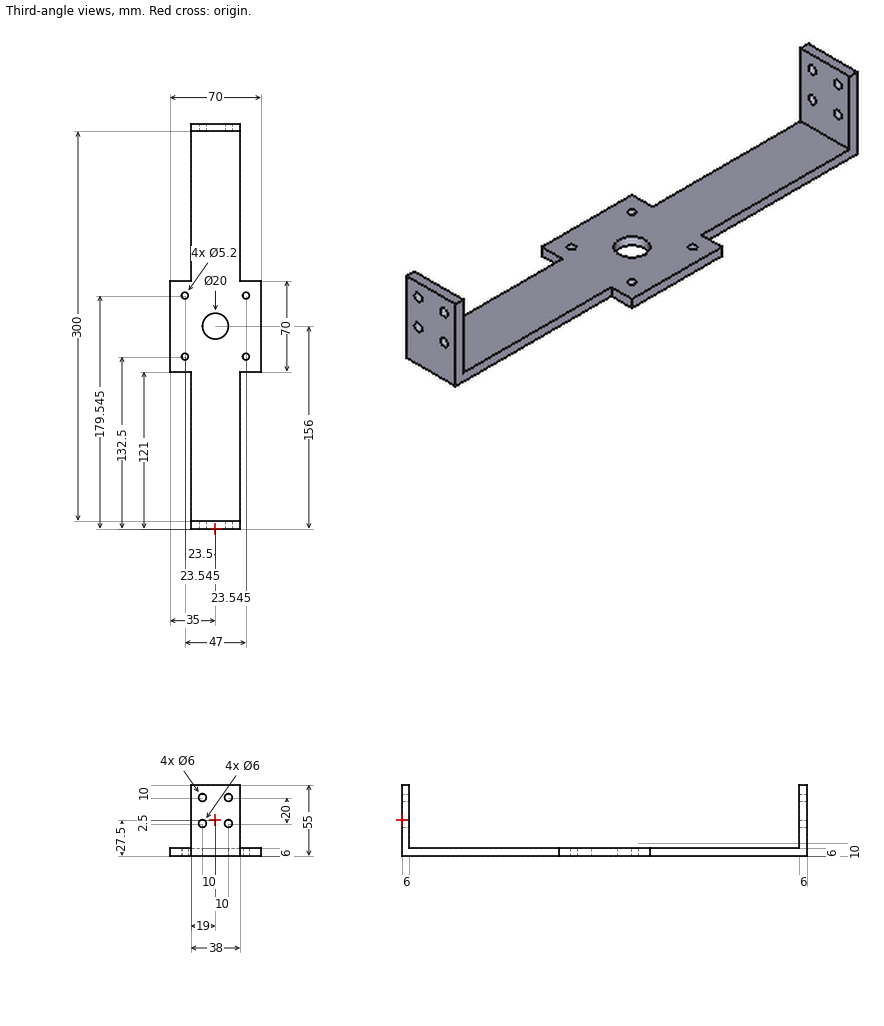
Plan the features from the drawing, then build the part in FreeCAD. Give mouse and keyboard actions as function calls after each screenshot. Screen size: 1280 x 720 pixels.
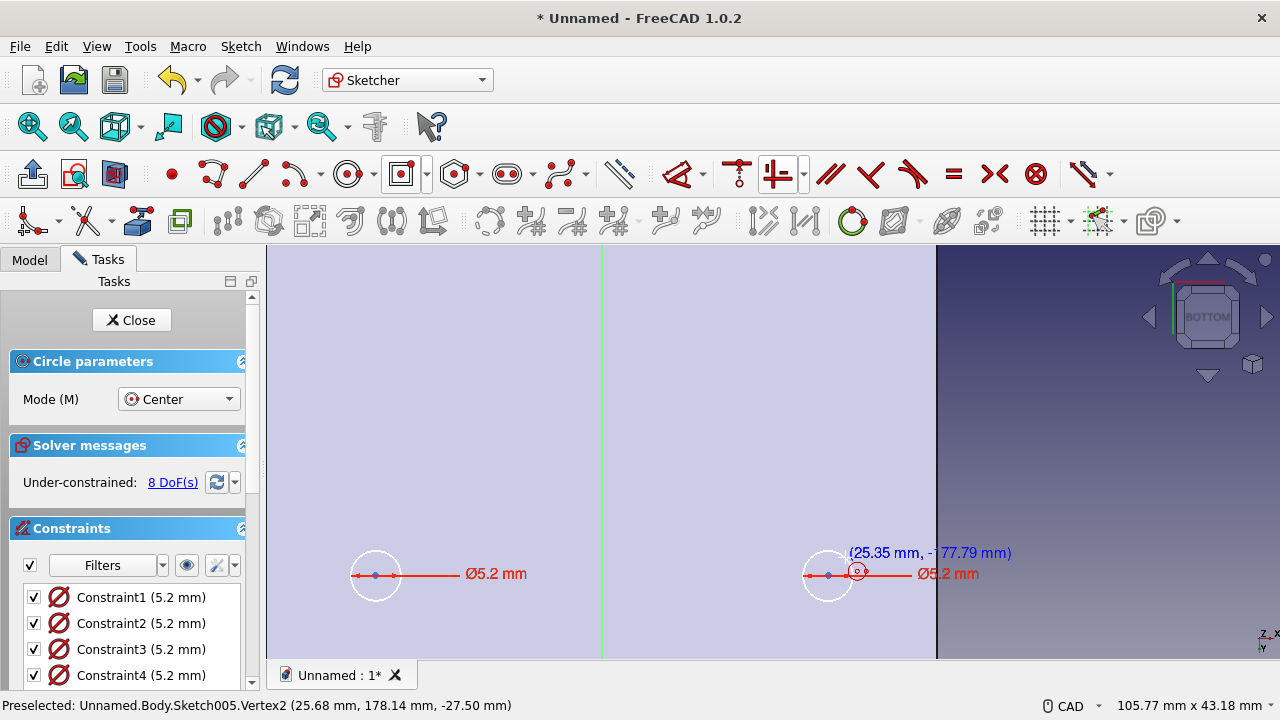
click(602, 349)
move(670, 281)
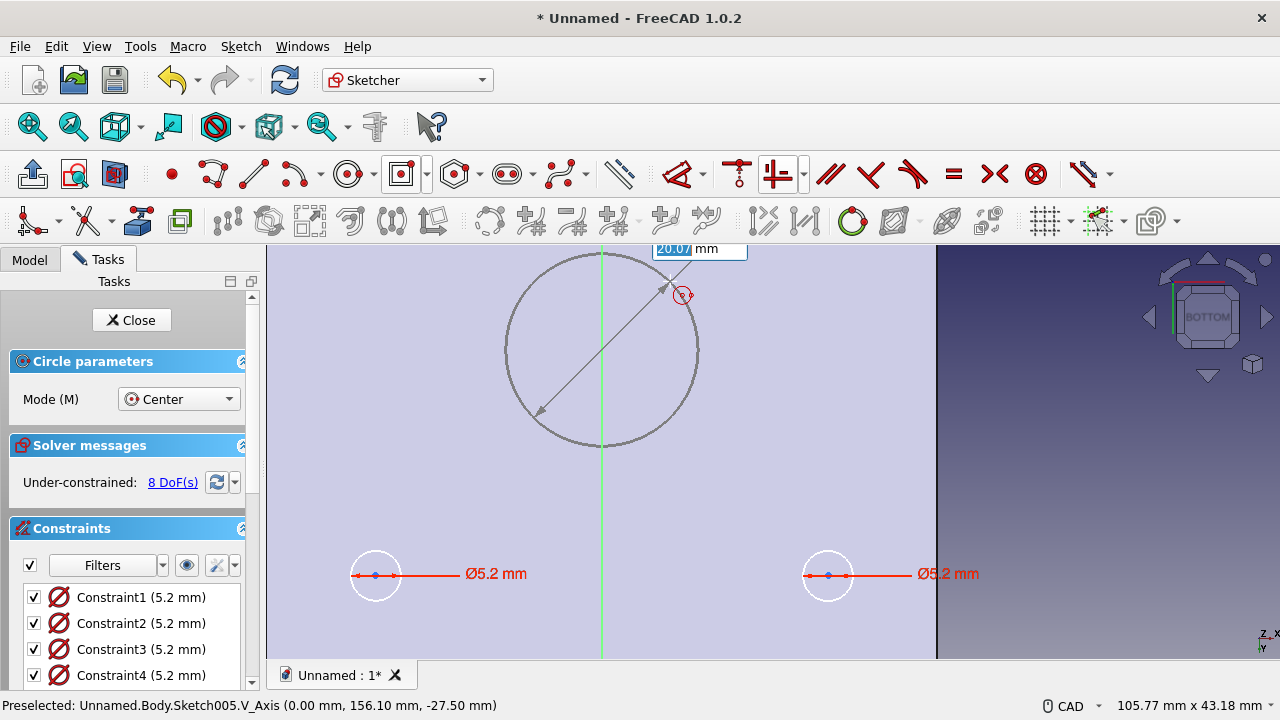
text(20)
key(Return)
key(Escape)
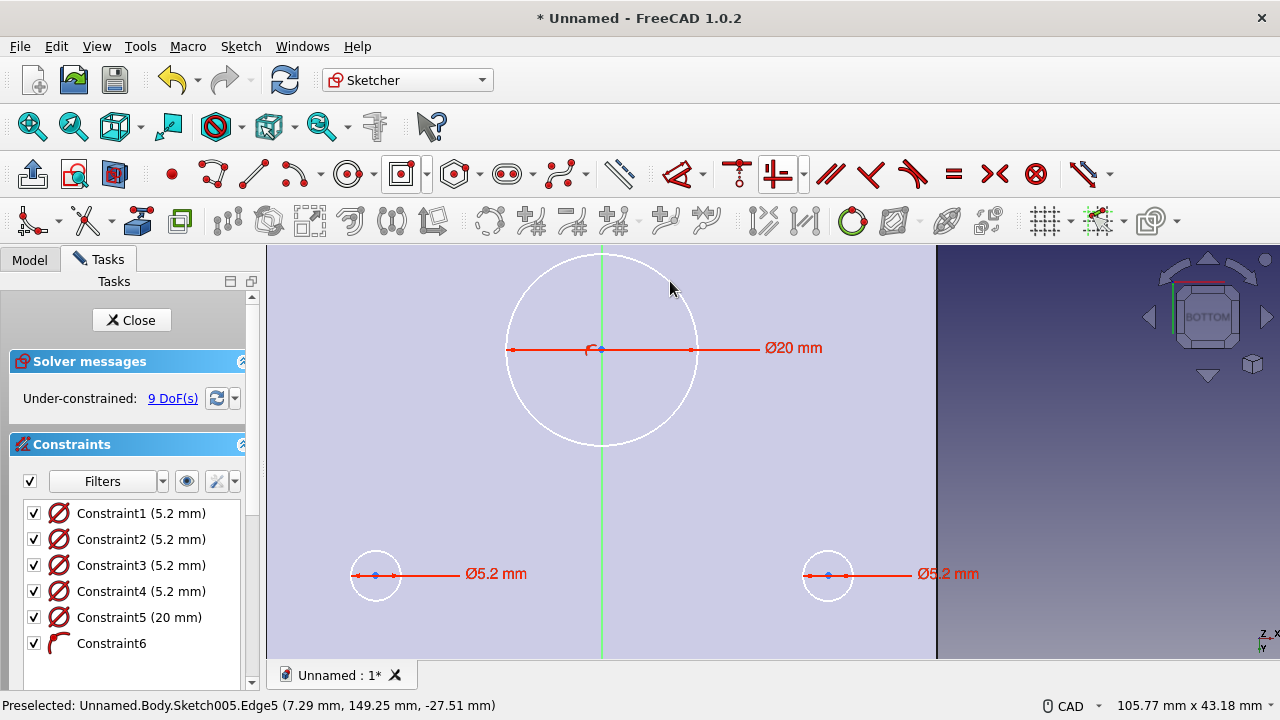
scroll(829, 577, down, 3)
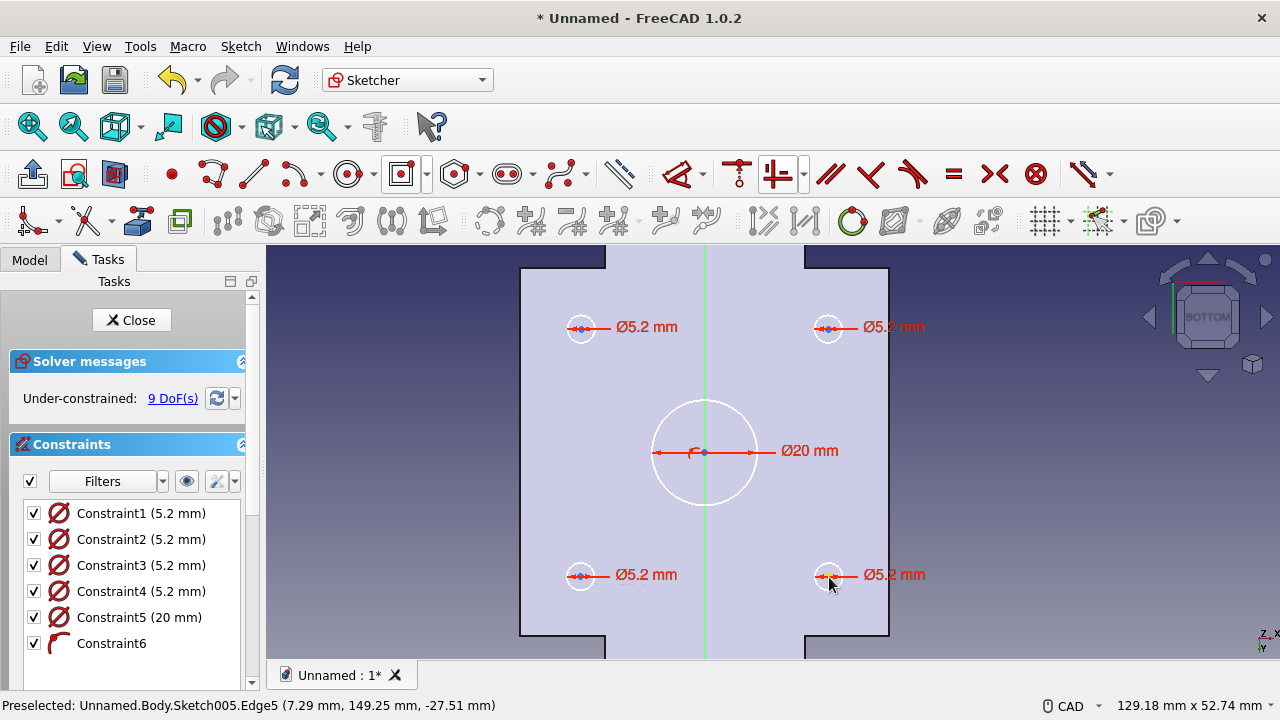
click(581, 329)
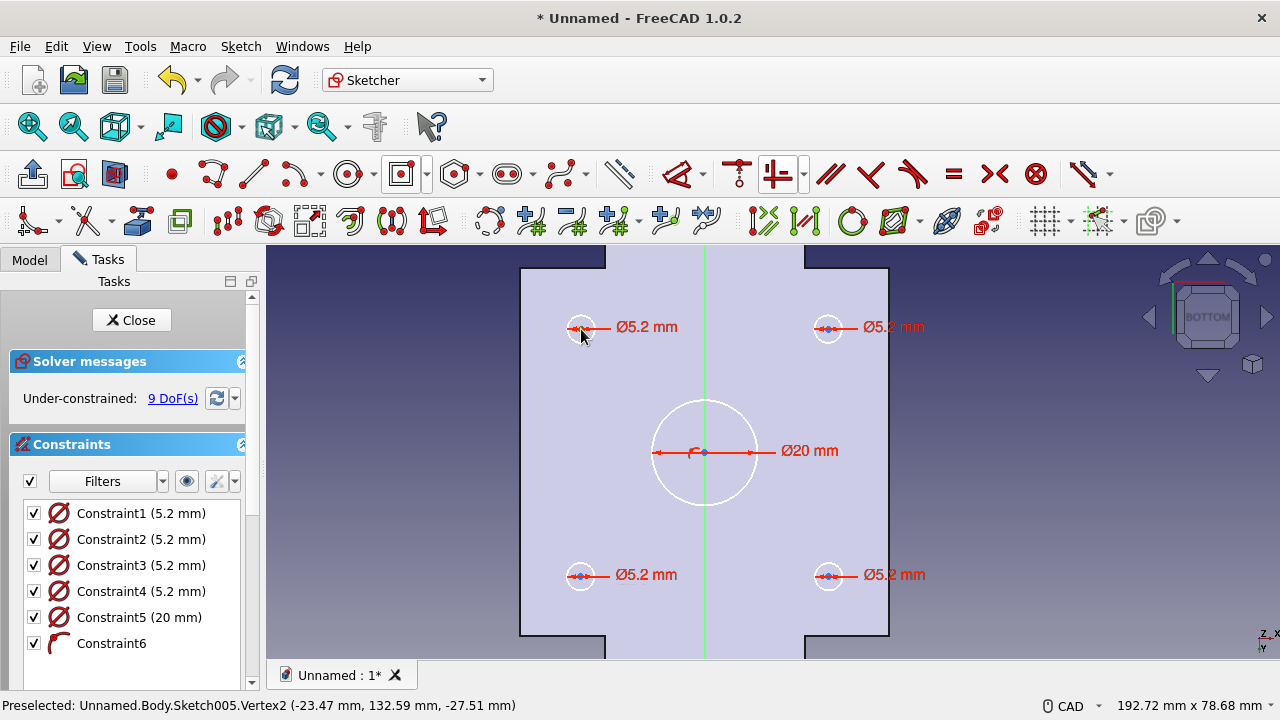
click(828, 329)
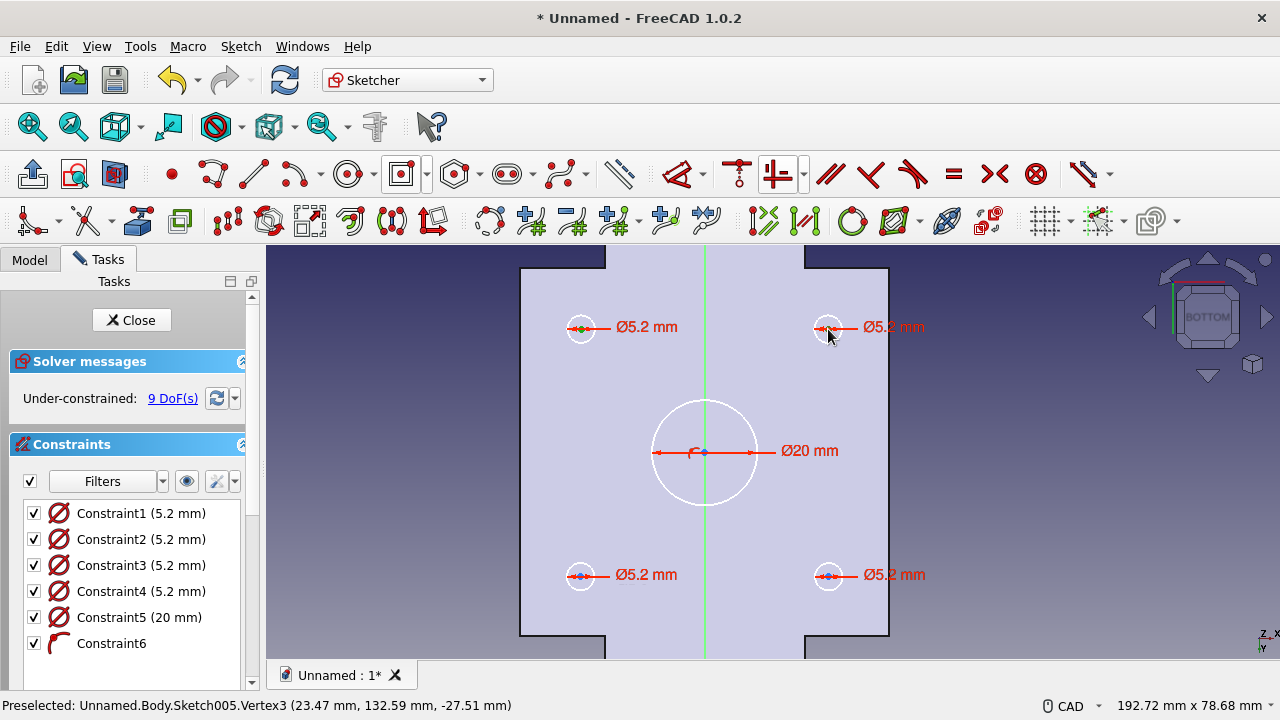
click(804, 174)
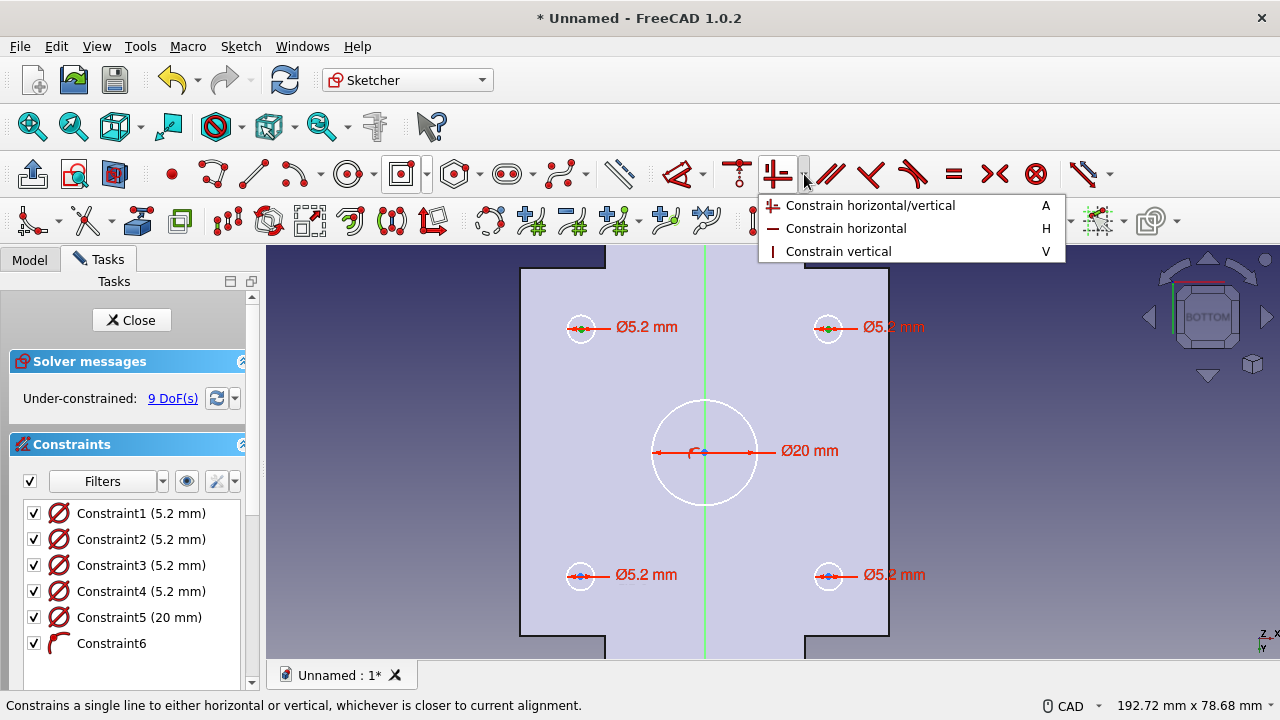
click(912, 228)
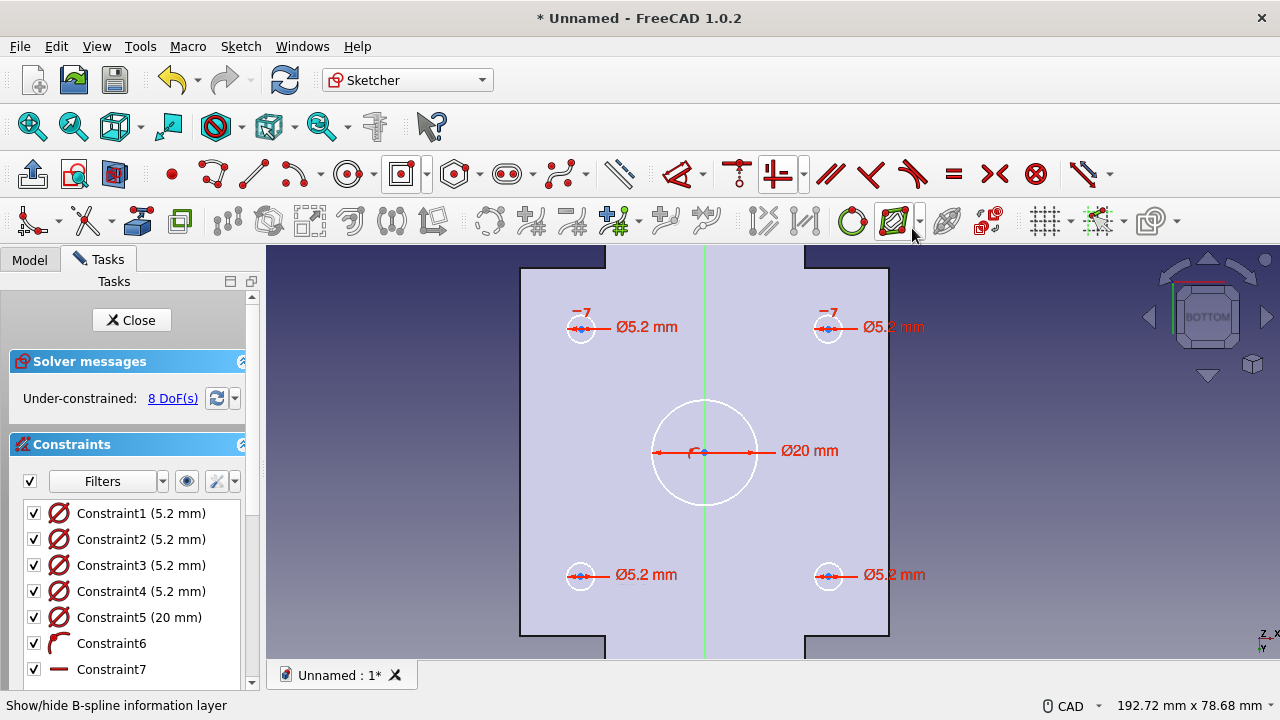
click(581, 577)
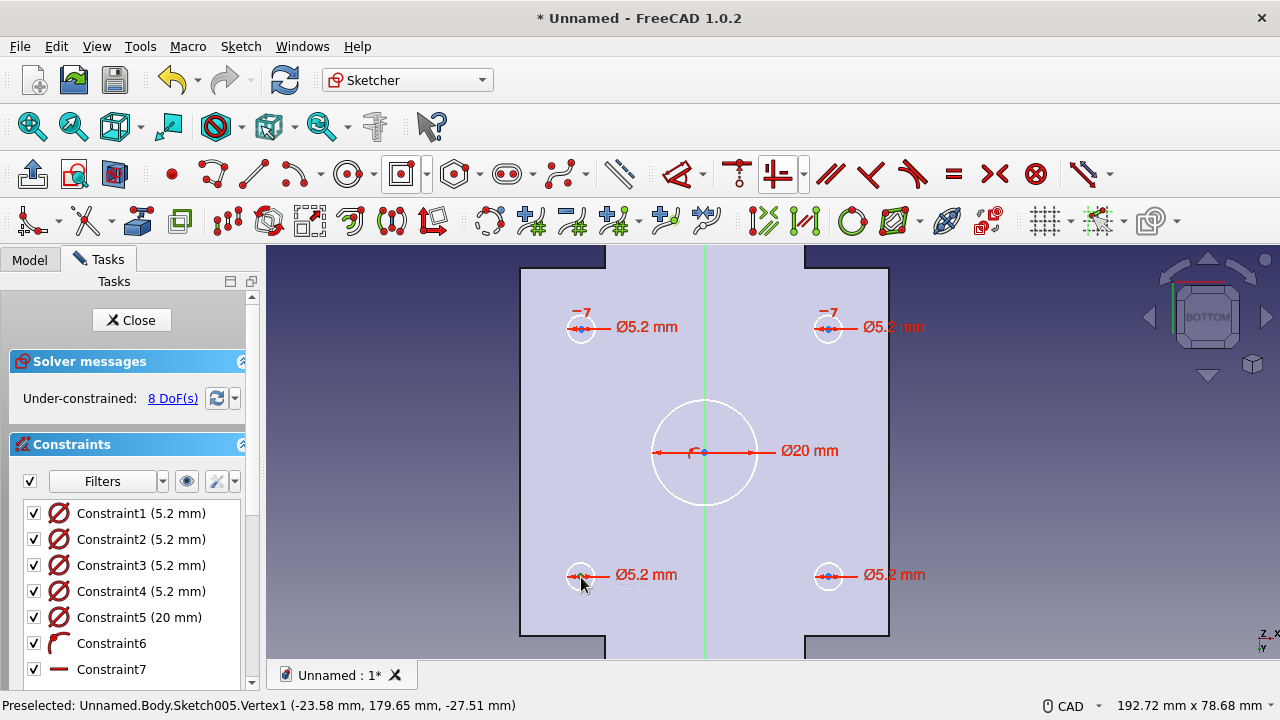
click(829, 577)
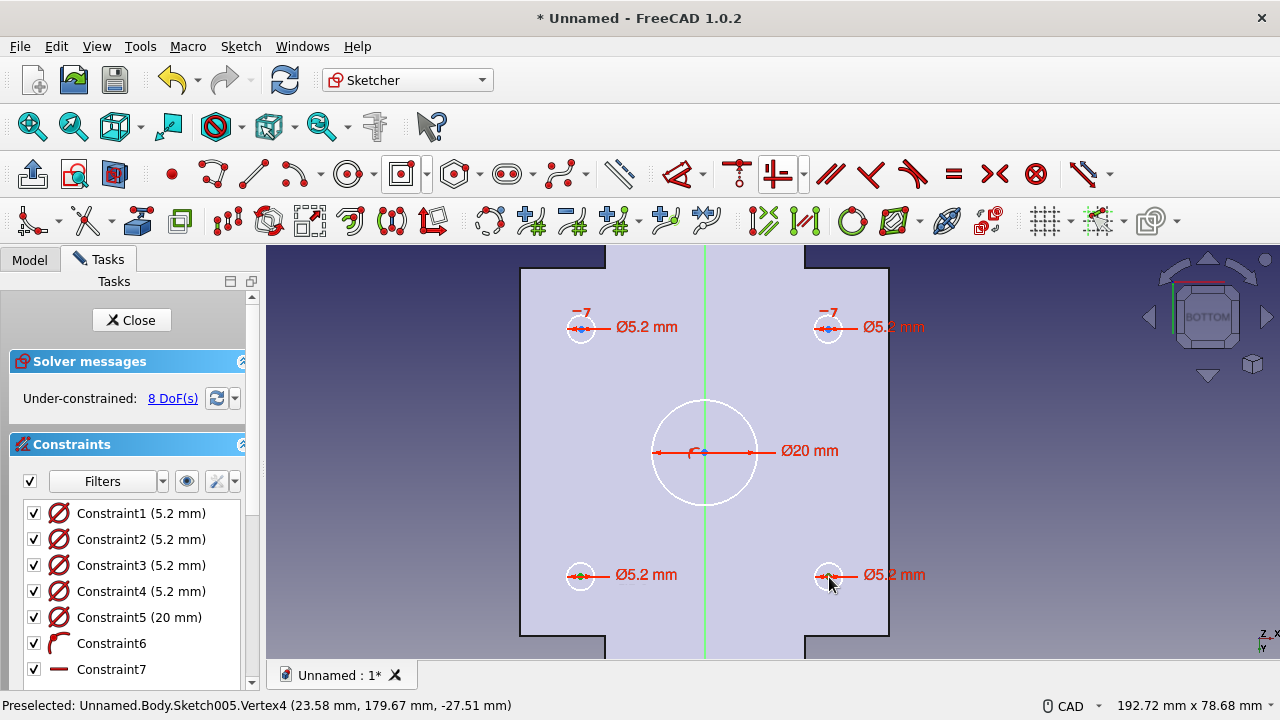
key(h)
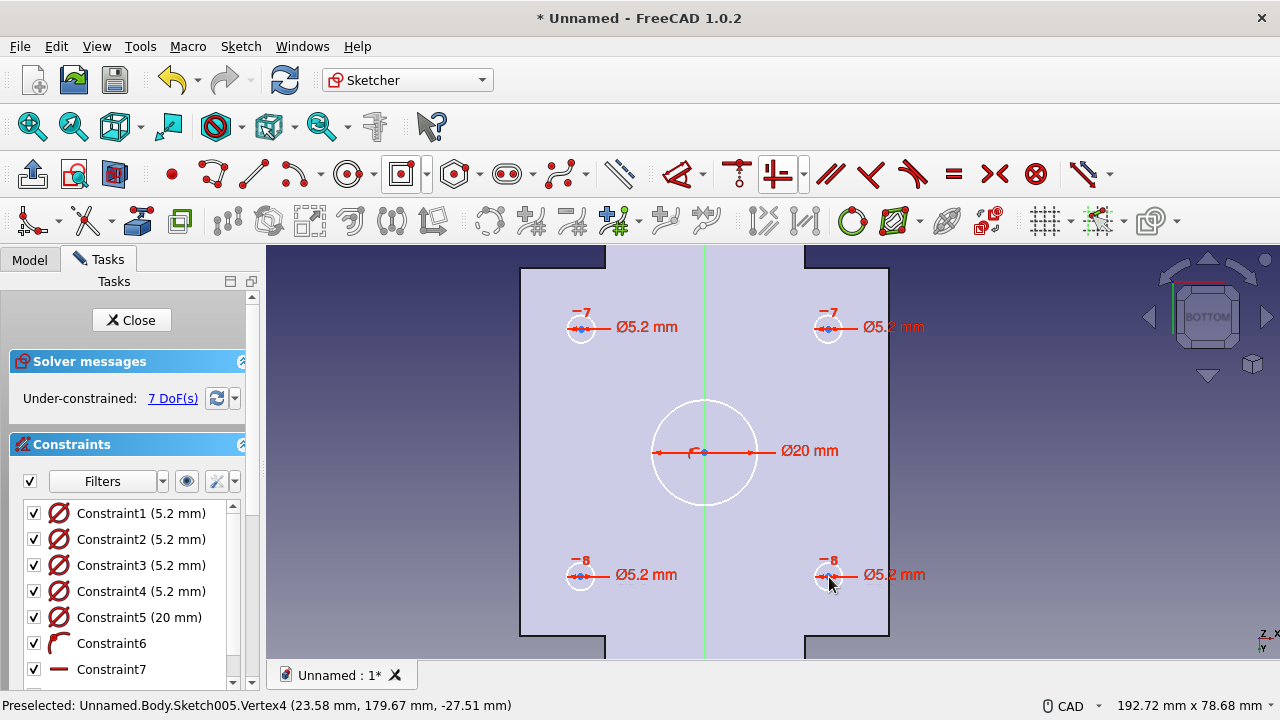
key(d)